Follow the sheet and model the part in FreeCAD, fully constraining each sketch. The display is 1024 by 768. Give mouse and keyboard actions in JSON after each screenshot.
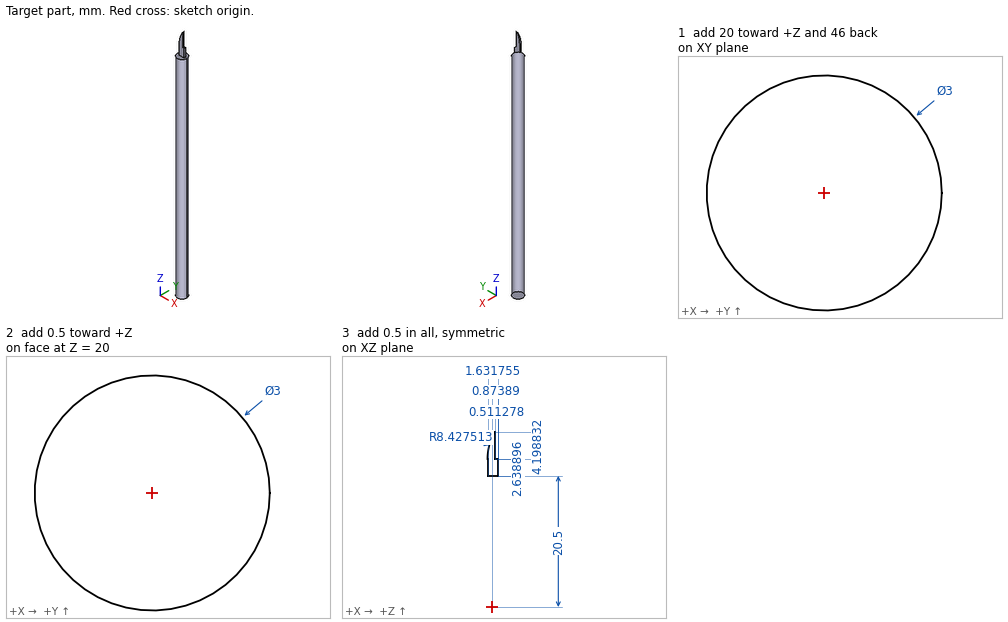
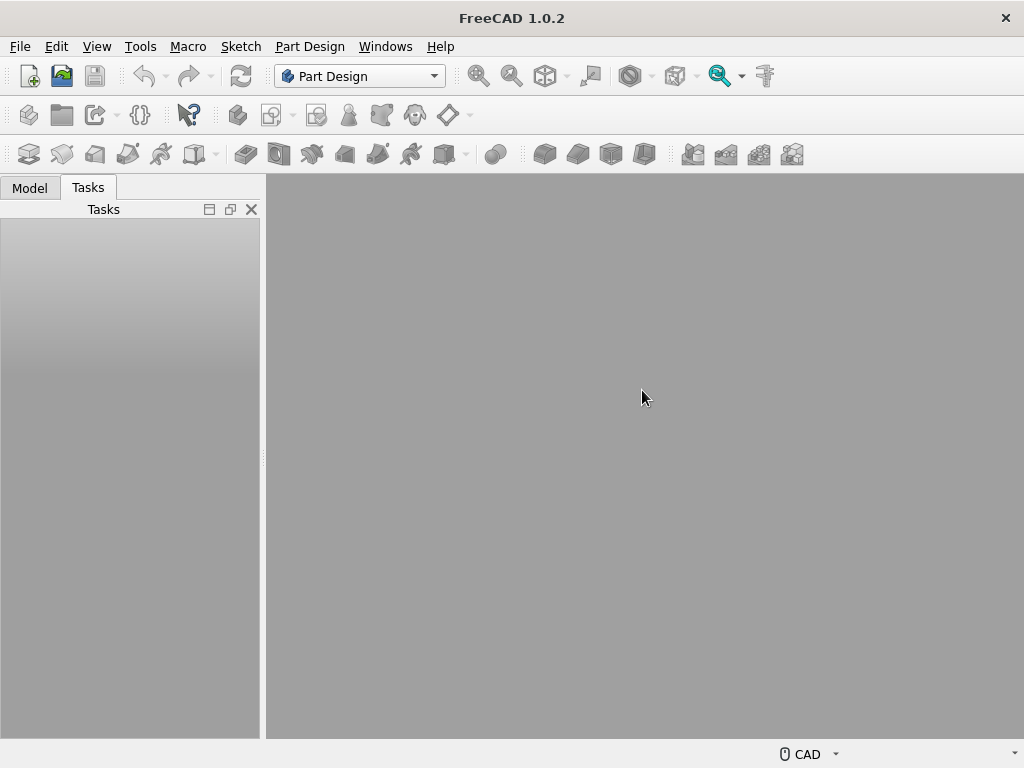
{"action": "left_click", "coordinate": [29, 76]}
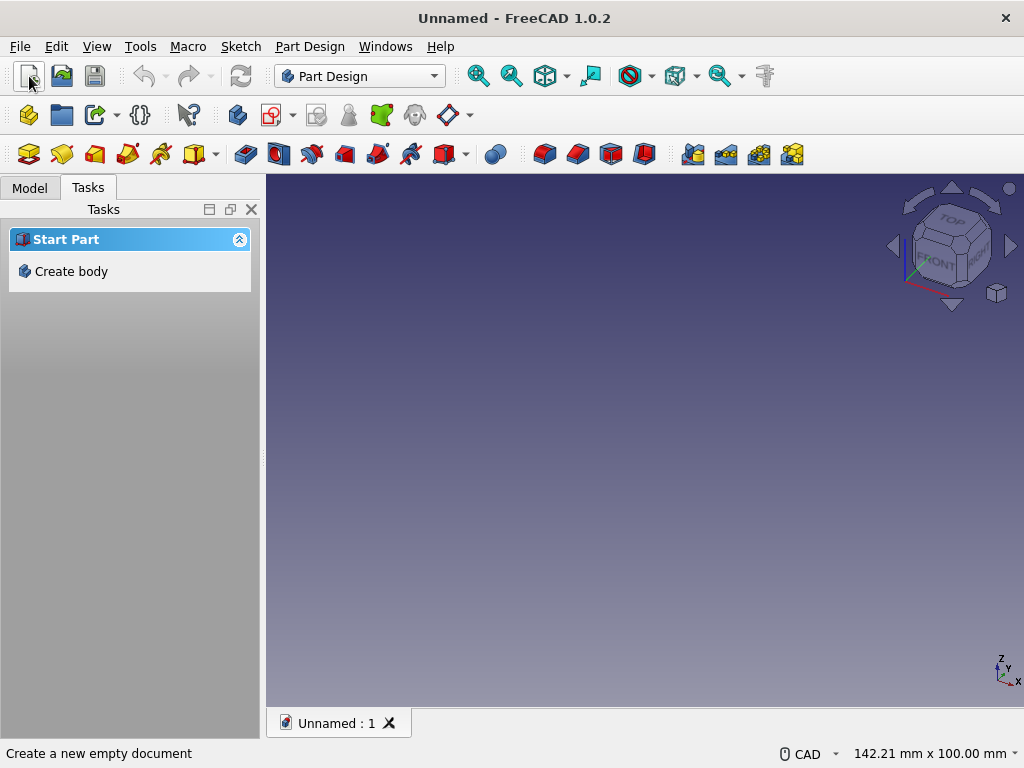
{"action": "left_click", "coordinate": [270, 116]}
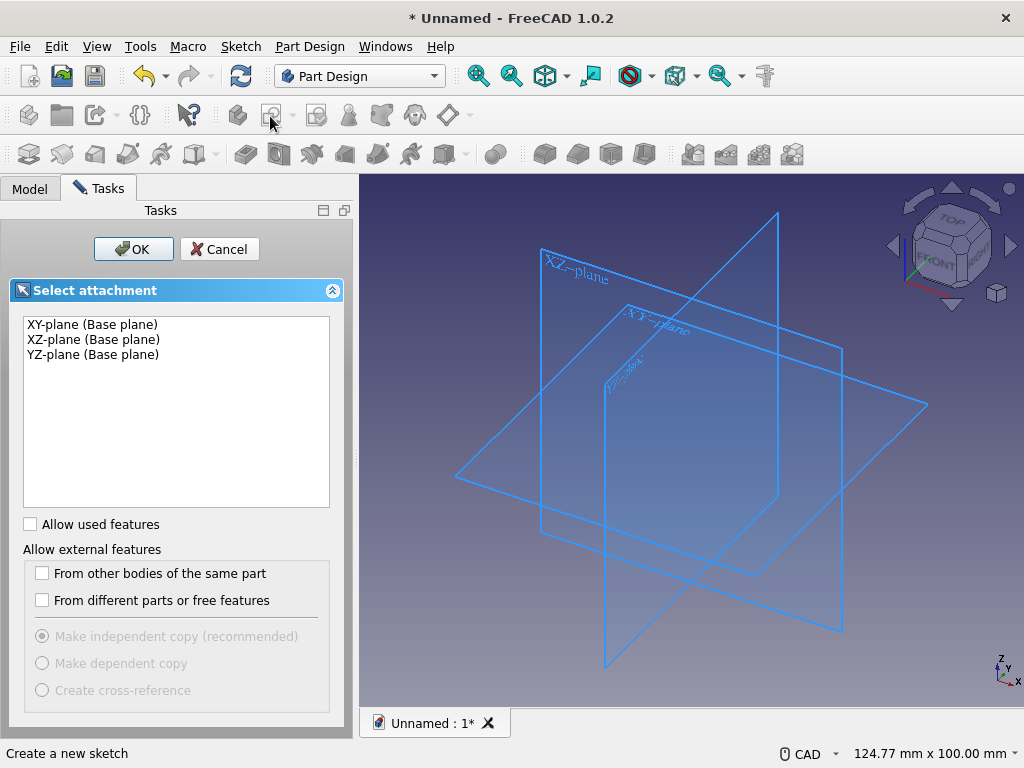
{"action": "left_click", "coordinate": [84, 324]}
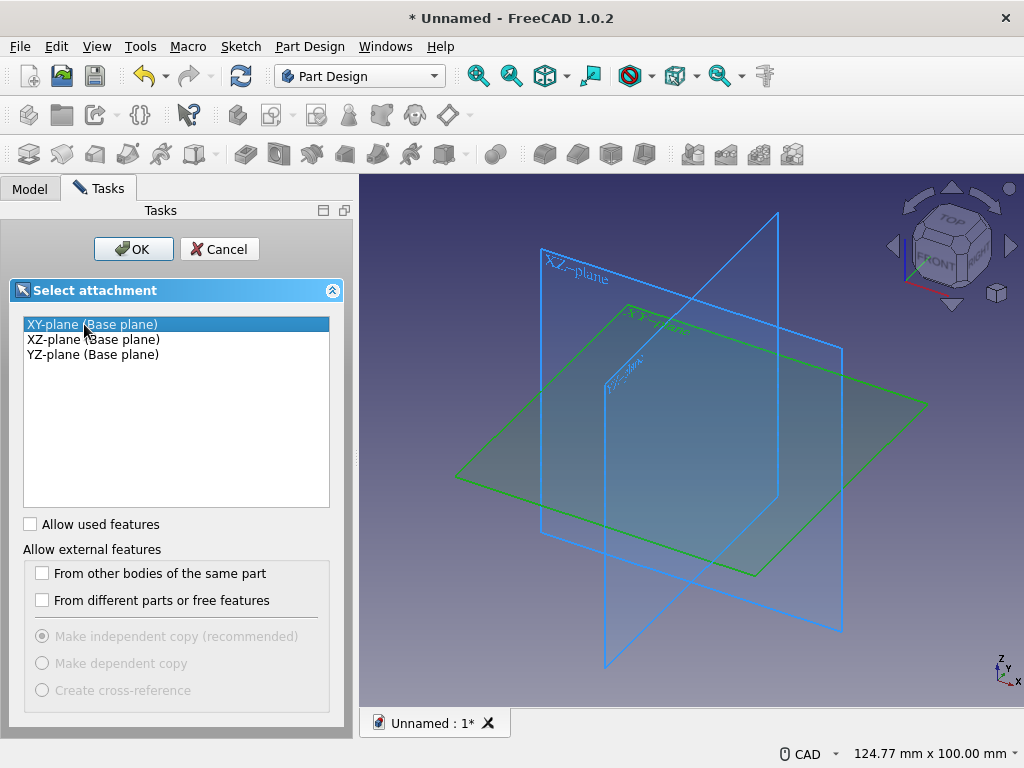
{"action": "left_click", "coordinate": [134, 249]}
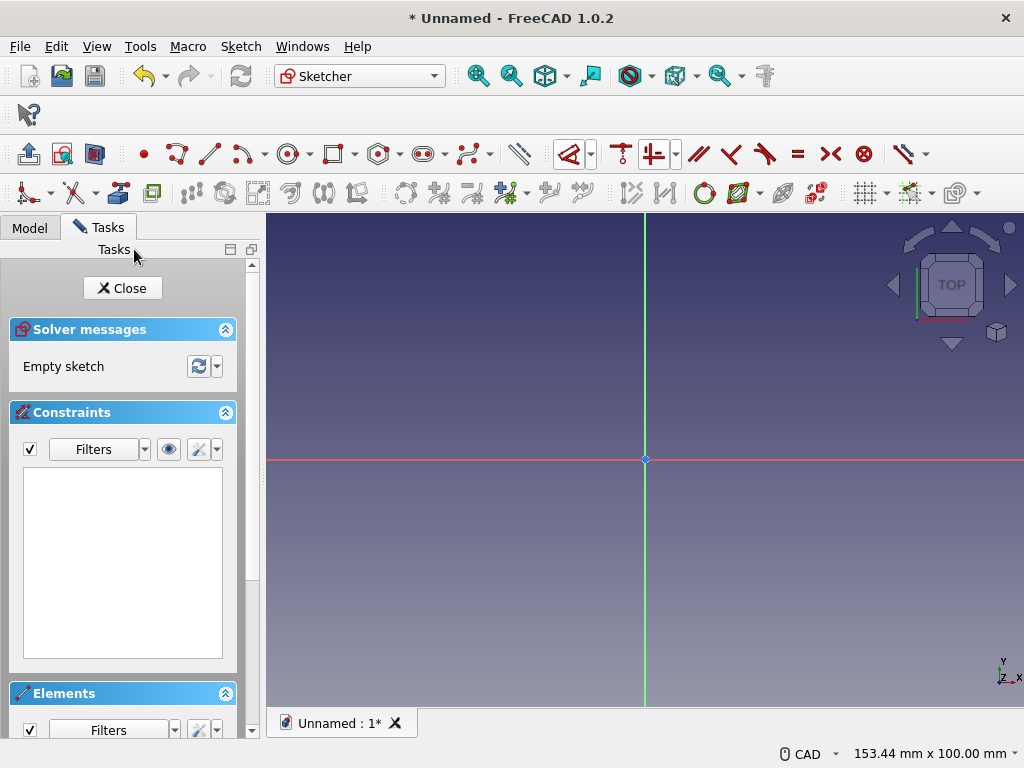
{"action": "scroll", "coordinate": [649, 460], "scroll_direction": "up", "scroll_amount": 15}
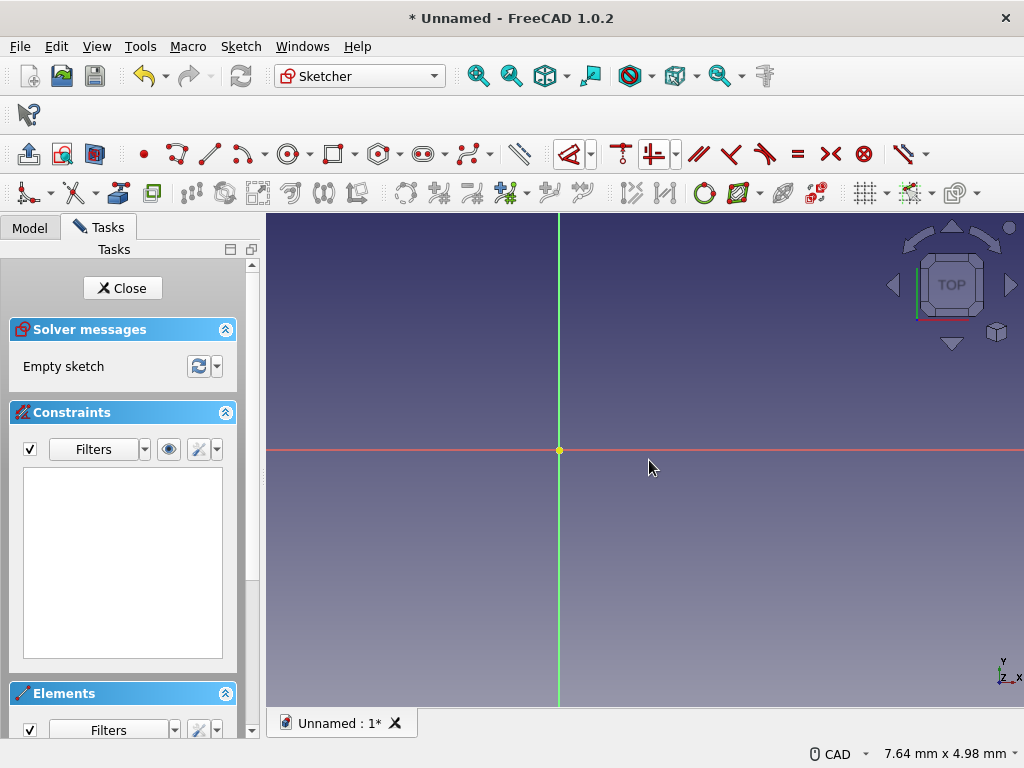
{"action": "left_click", "coordinate": [288, 154]}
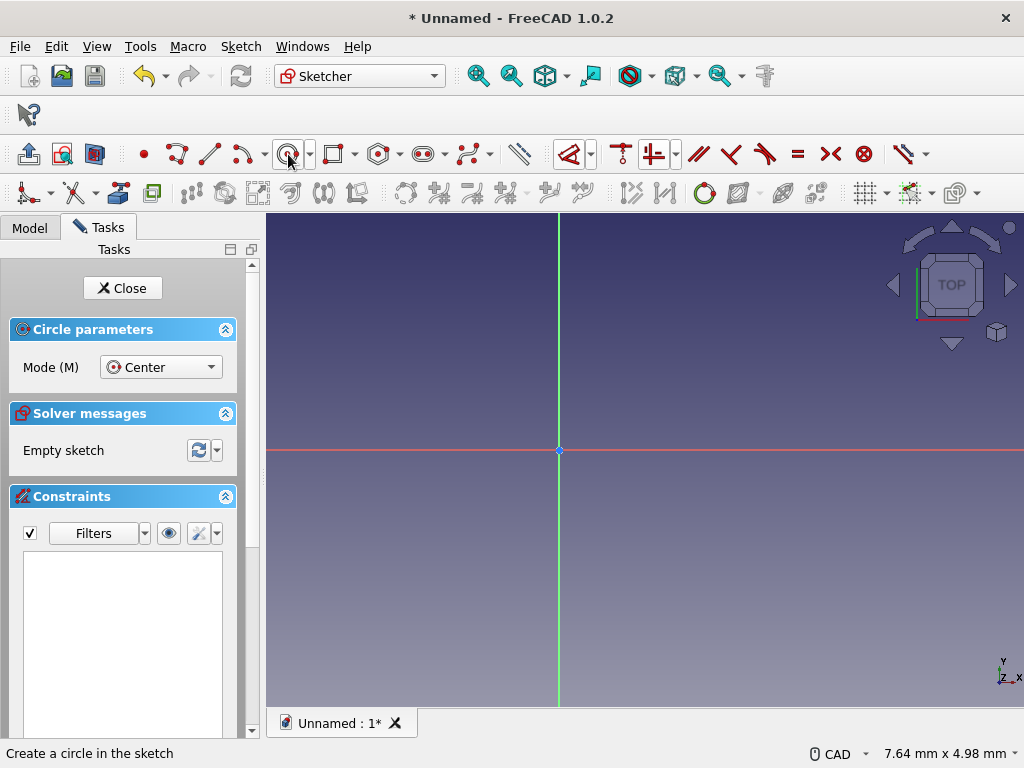
{"action": "left_click", "coordinate": [559, 450]}
{"action": "mouse_move", "coordinate": [664, 345]}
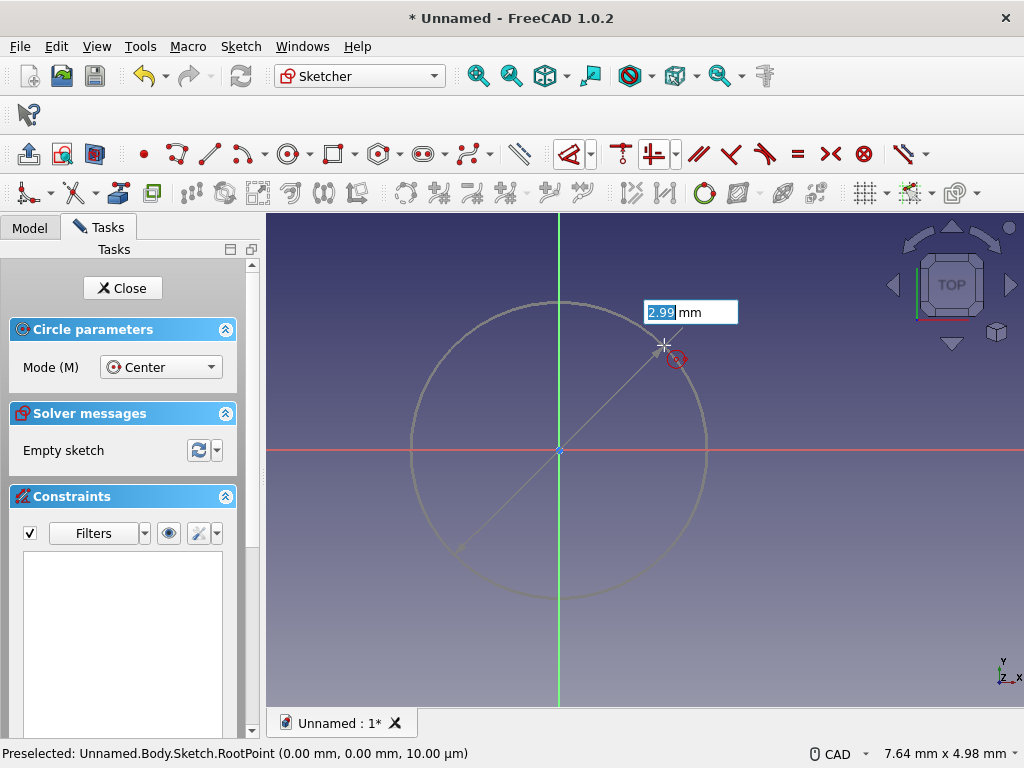
{"action": "type", "text": "3"}
{"action": "key", "text": "Return"}
{"action": "key", "text": "Escape"}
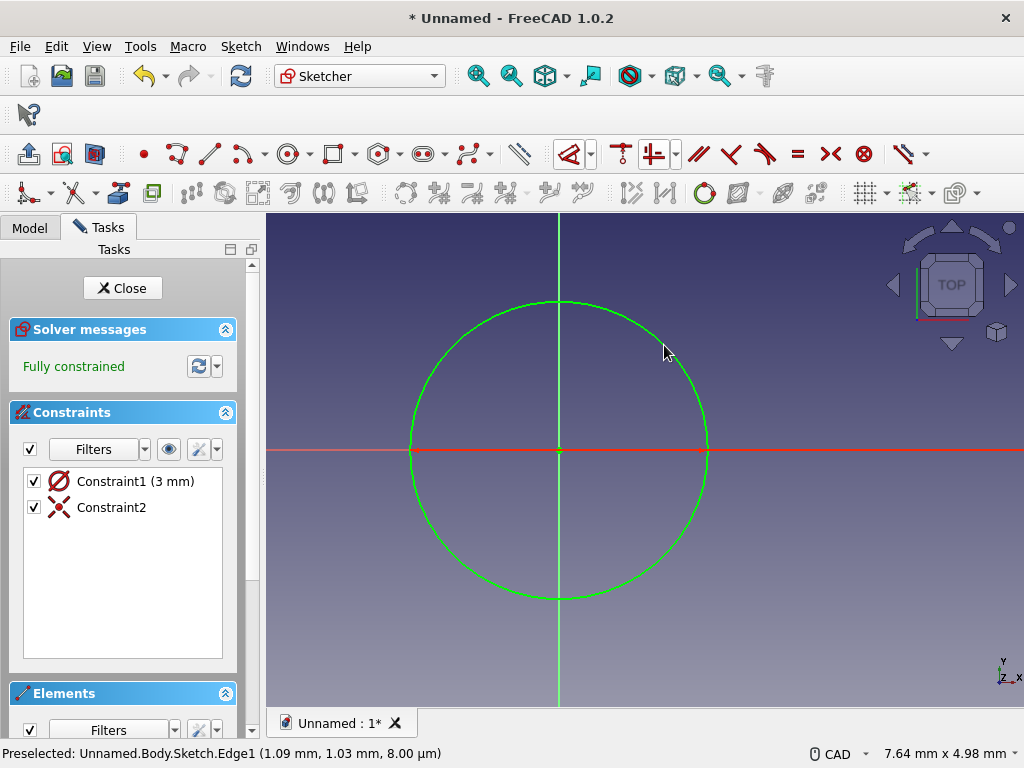
{"action": "left_click", "coordinate": [123, 288]}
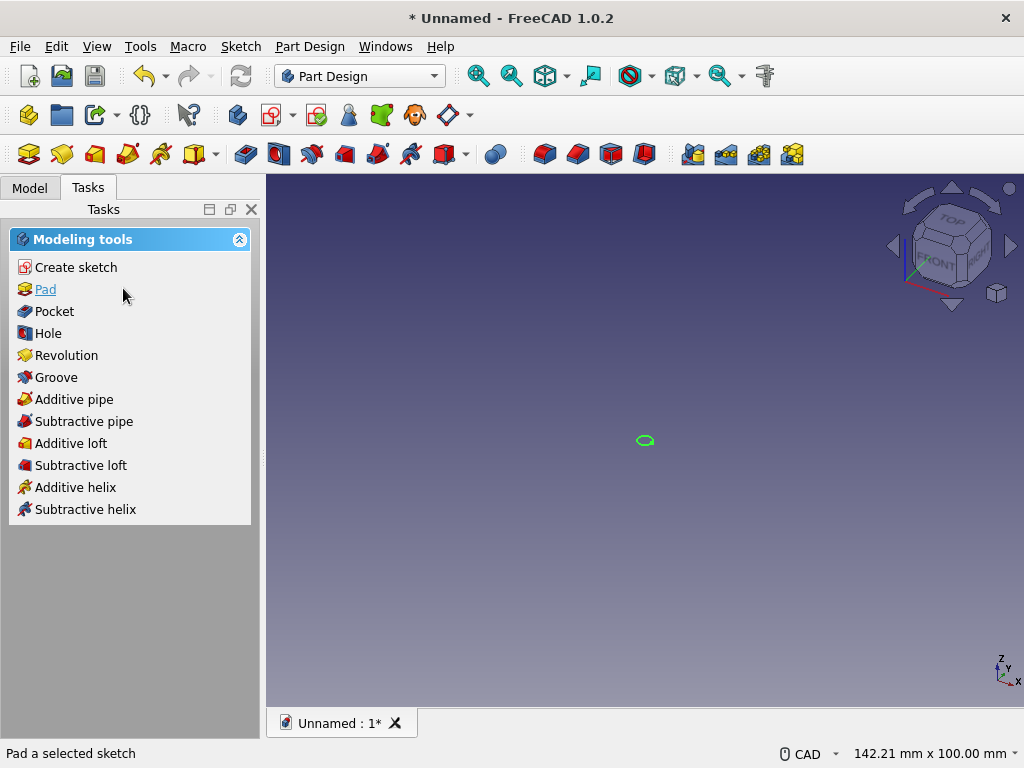
{"action": "left_click", "coordinate": [29, 154]}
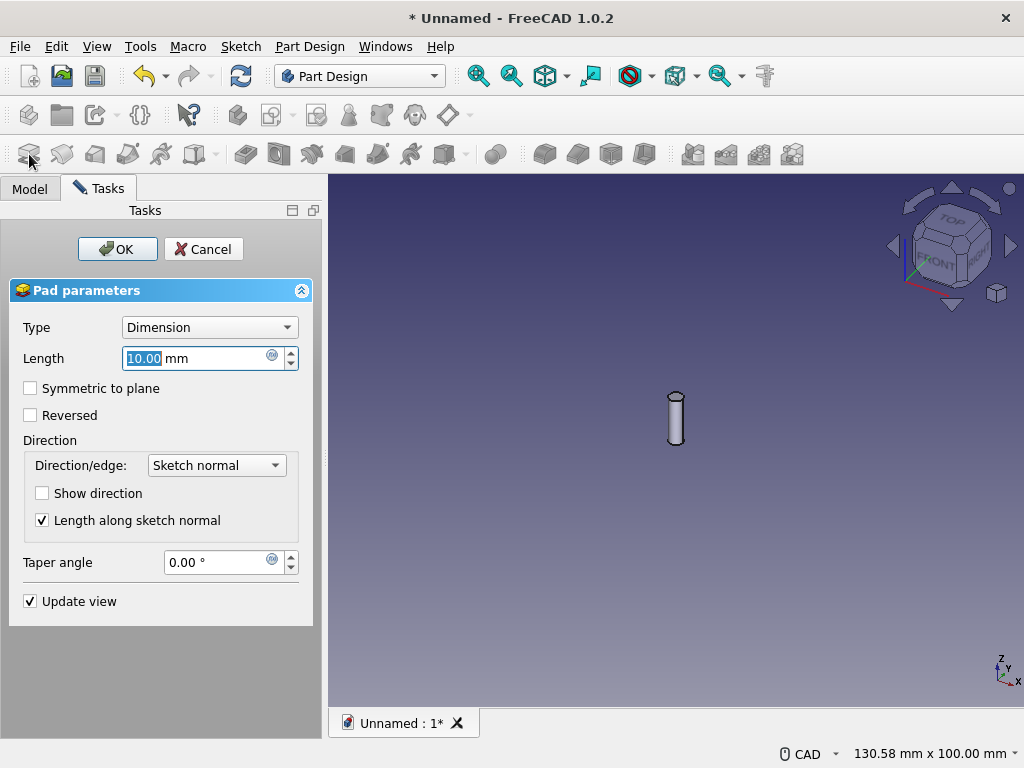
{"action": "left_click", "coordinate": [210, 328]}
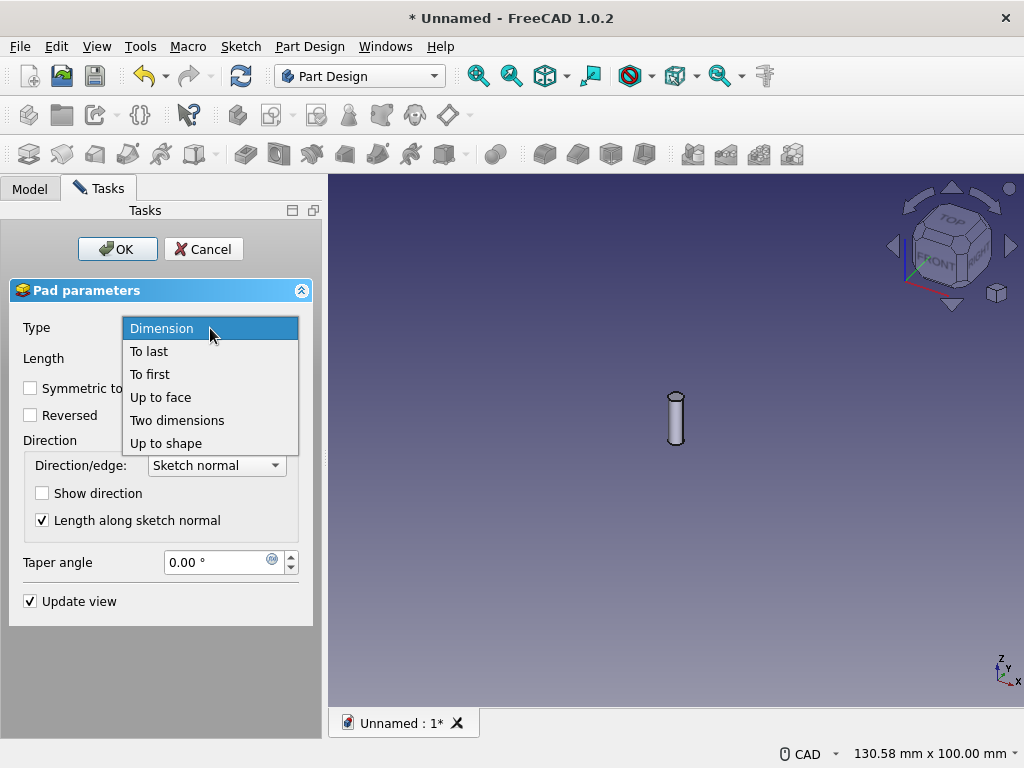
{"action": "left_click", "coordinate": [208, 420]}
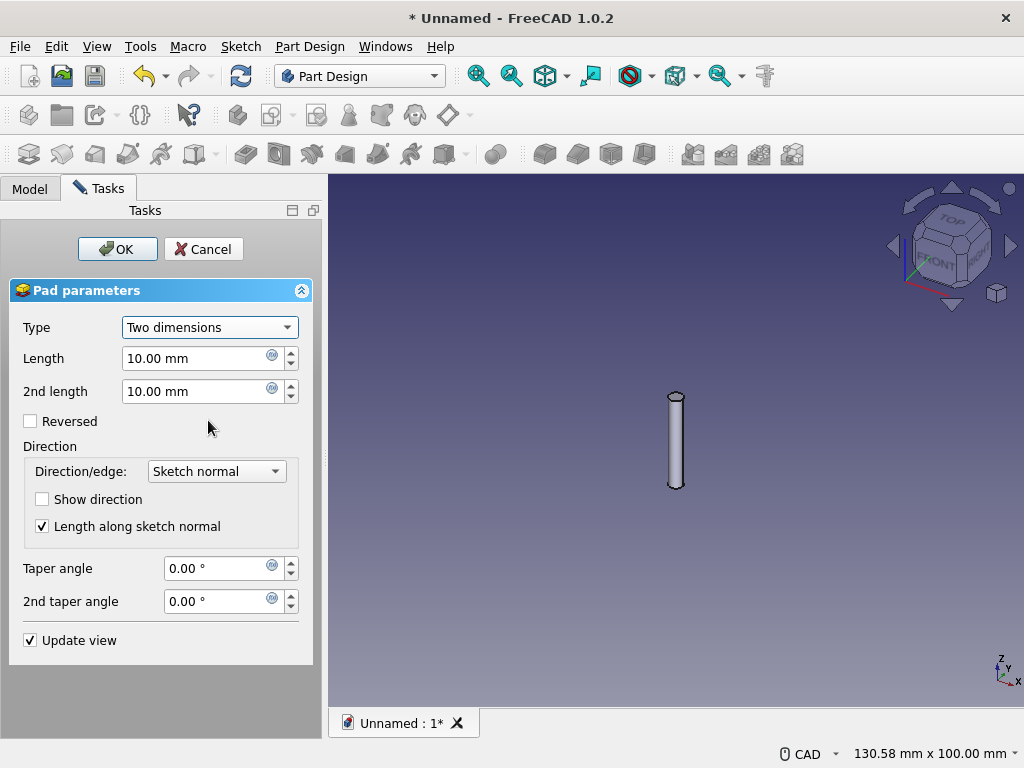
{"action": "triple_click", "coordinate": [204, 358]}